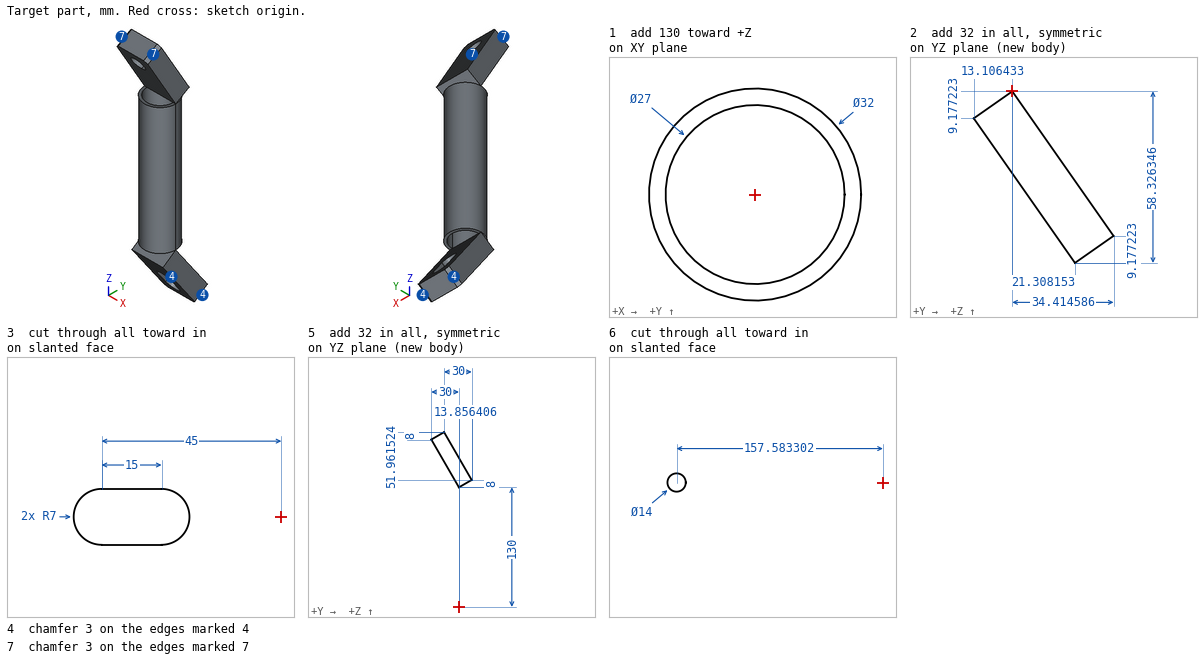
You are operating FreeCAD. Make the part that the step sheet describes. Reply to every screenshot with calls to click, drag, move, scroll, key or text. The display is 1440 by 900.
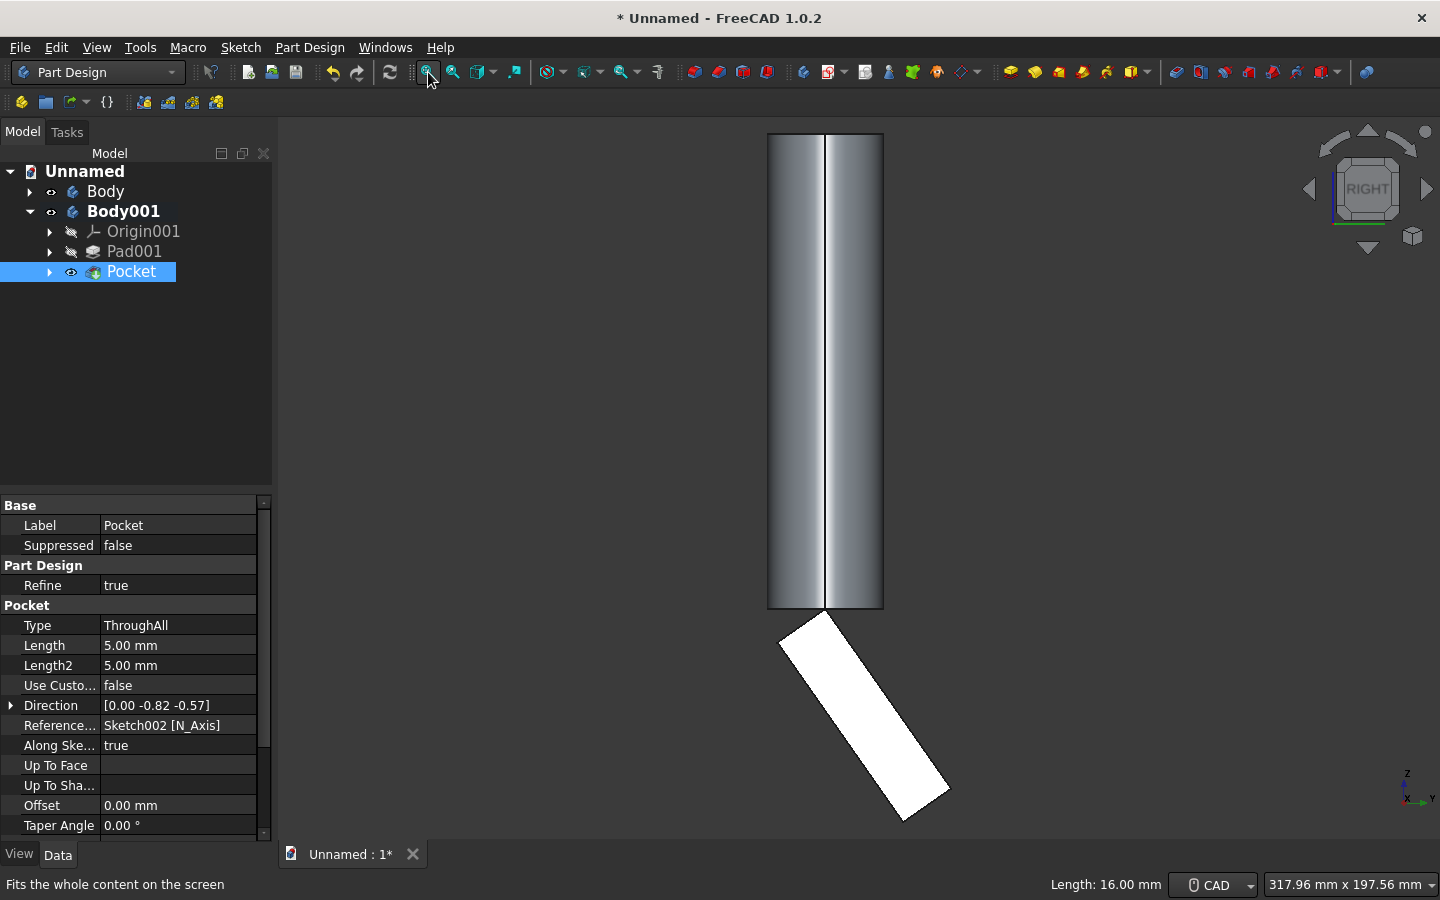
click(927, 804, ctrl)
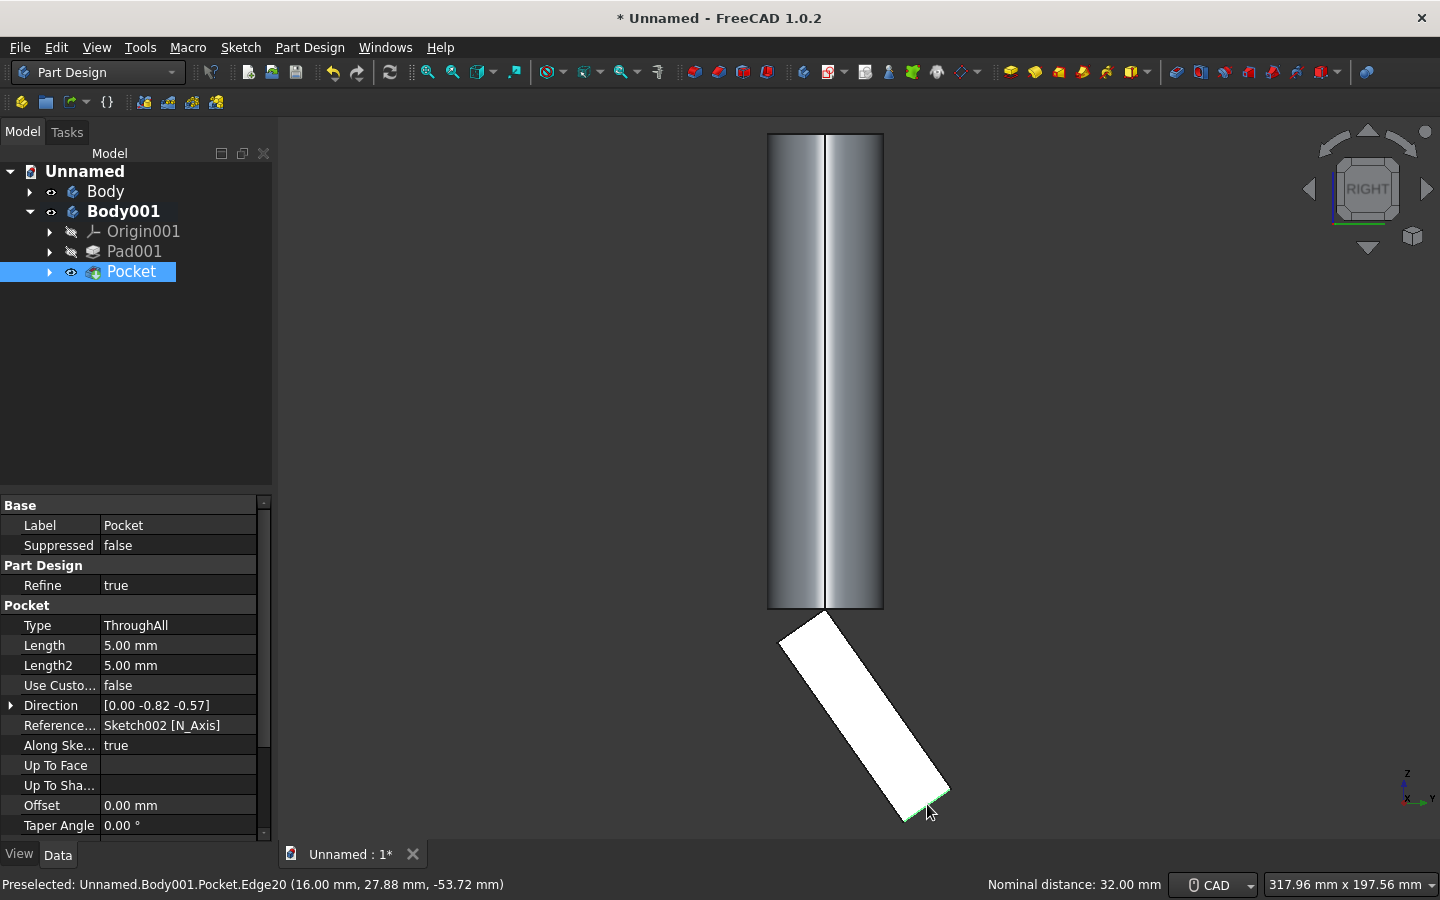
click(720, 72)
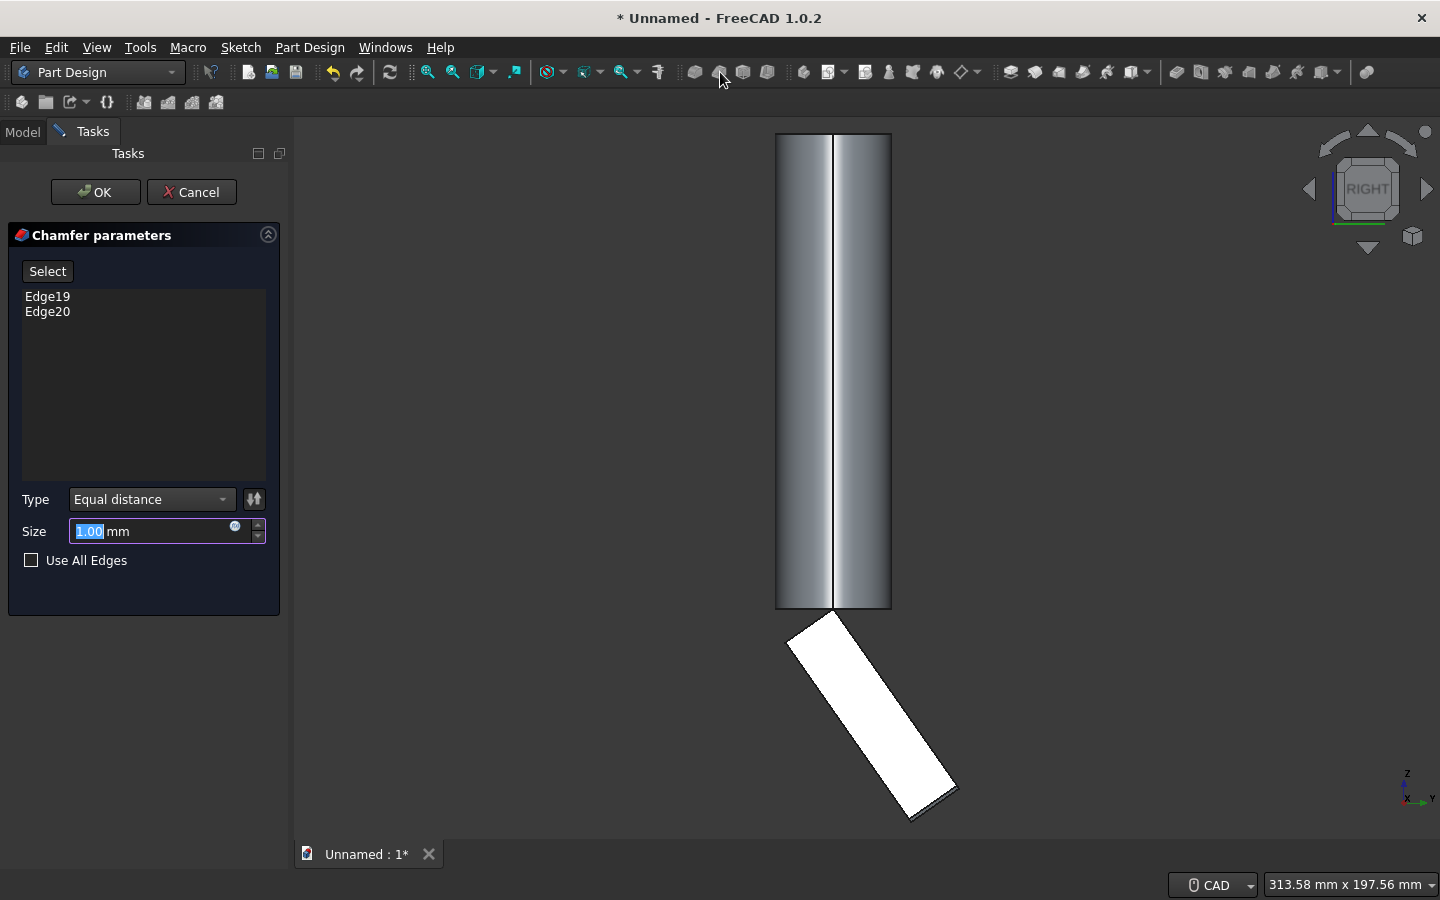
text(3)
key(Tab)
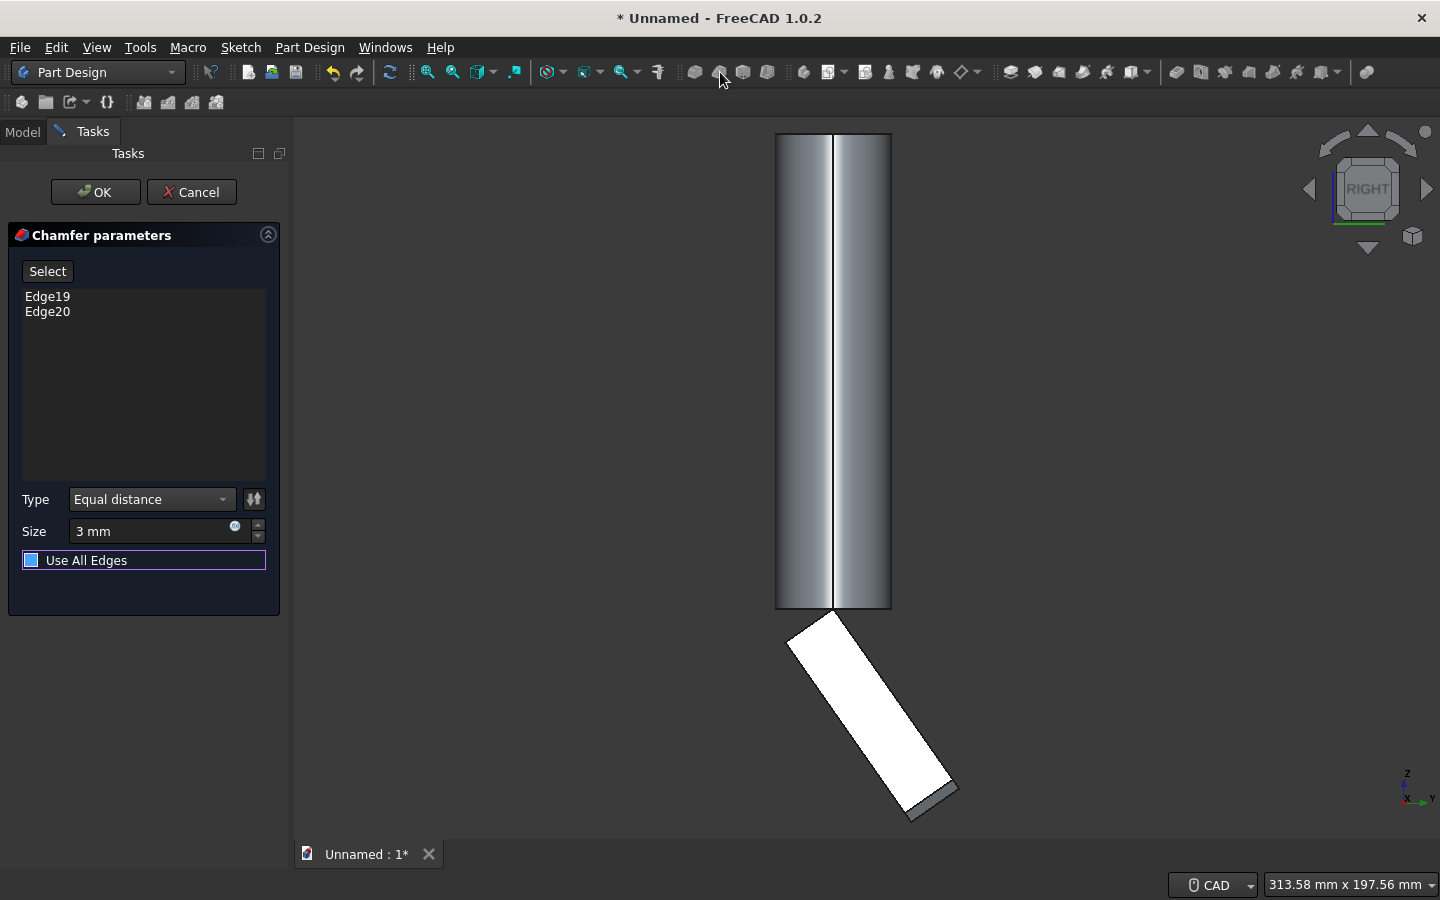
click(96, 192)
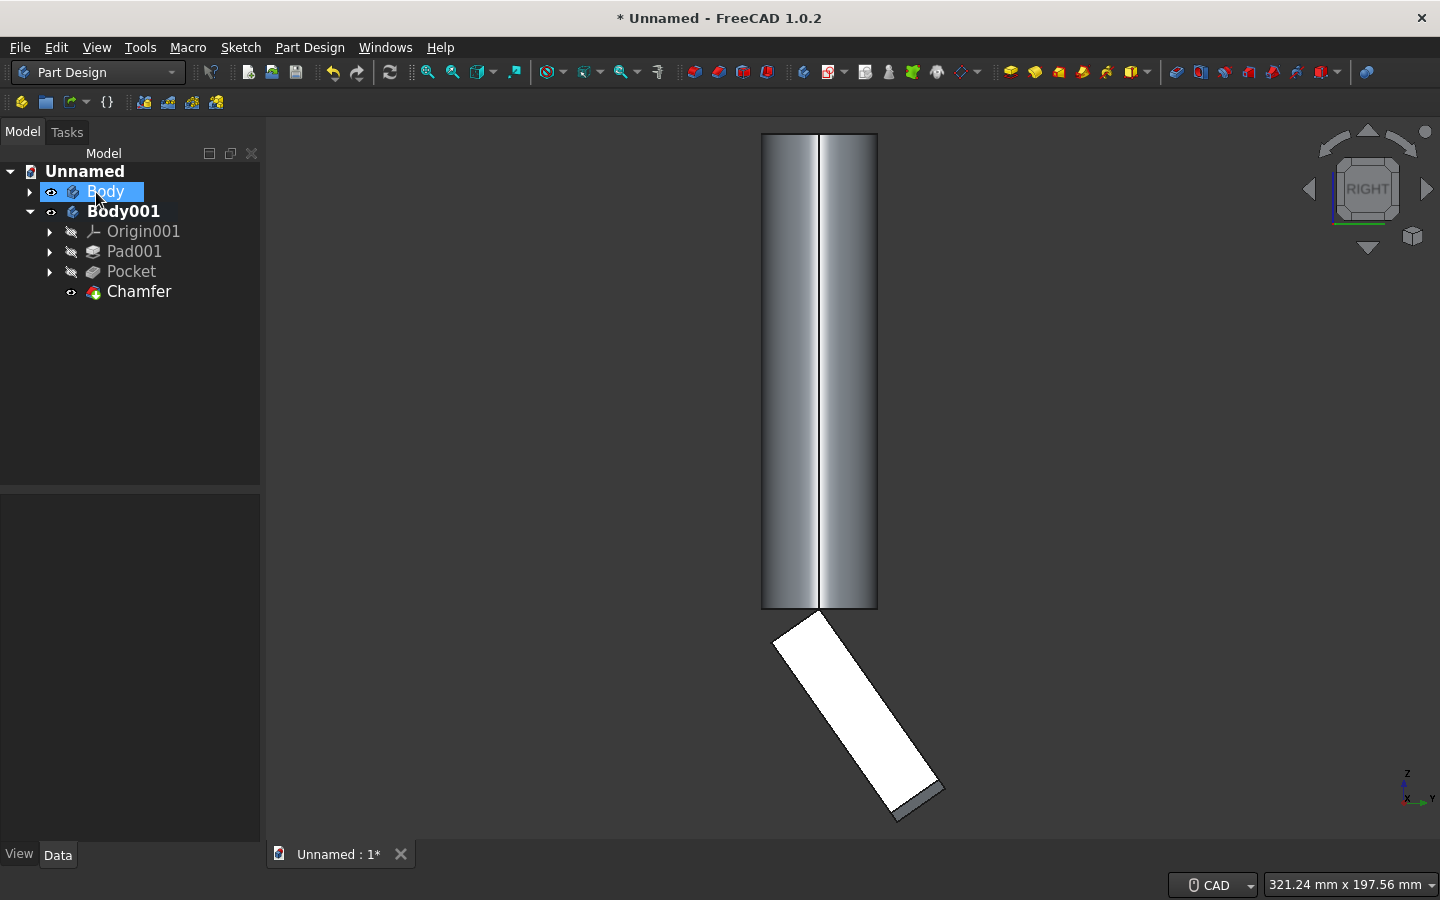
key(v)
key(f)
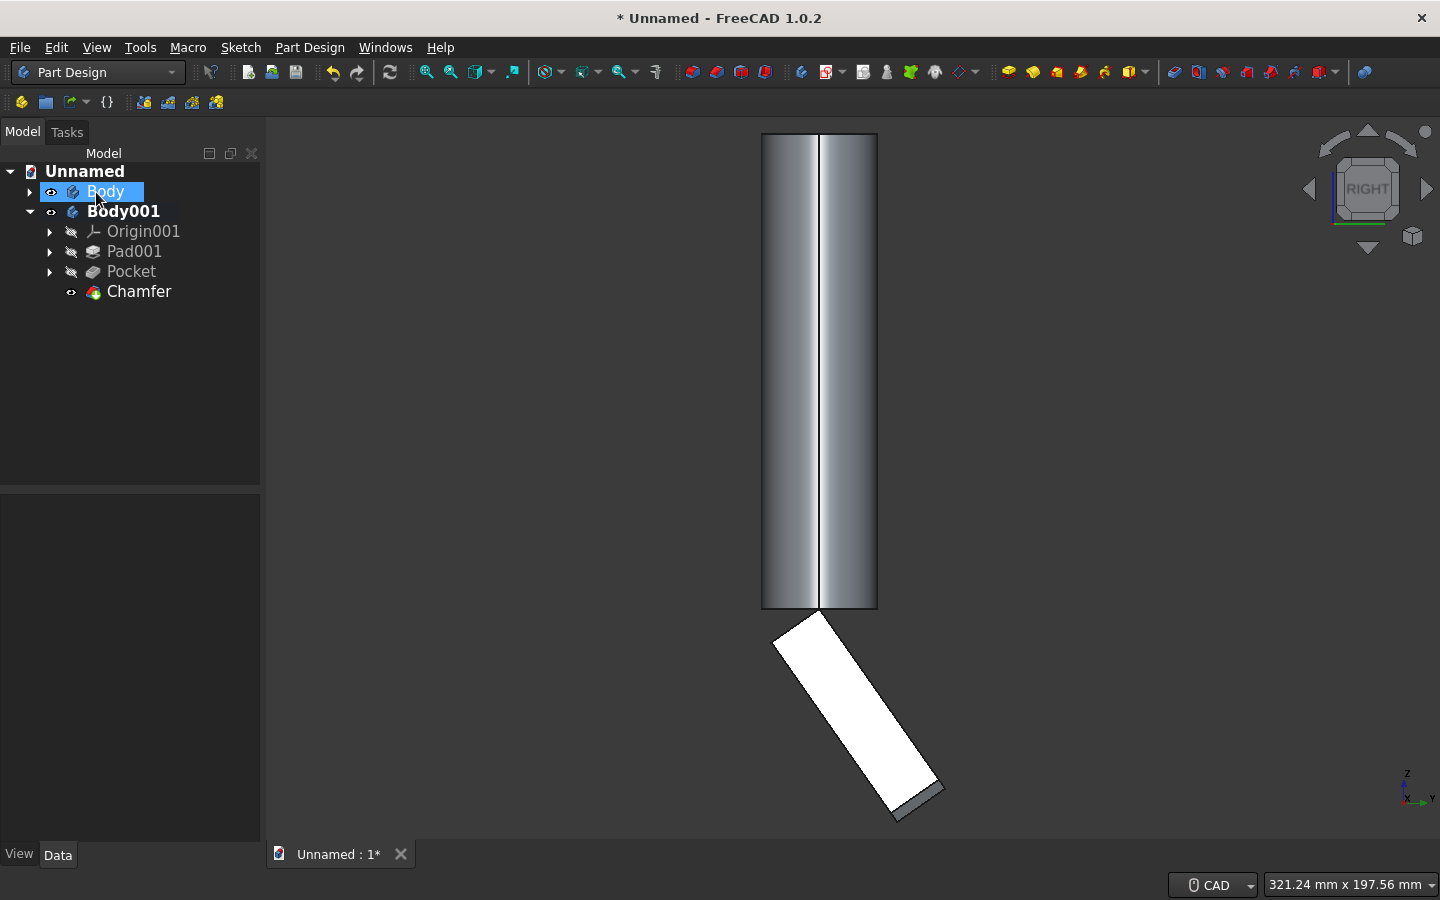
click(802, 72)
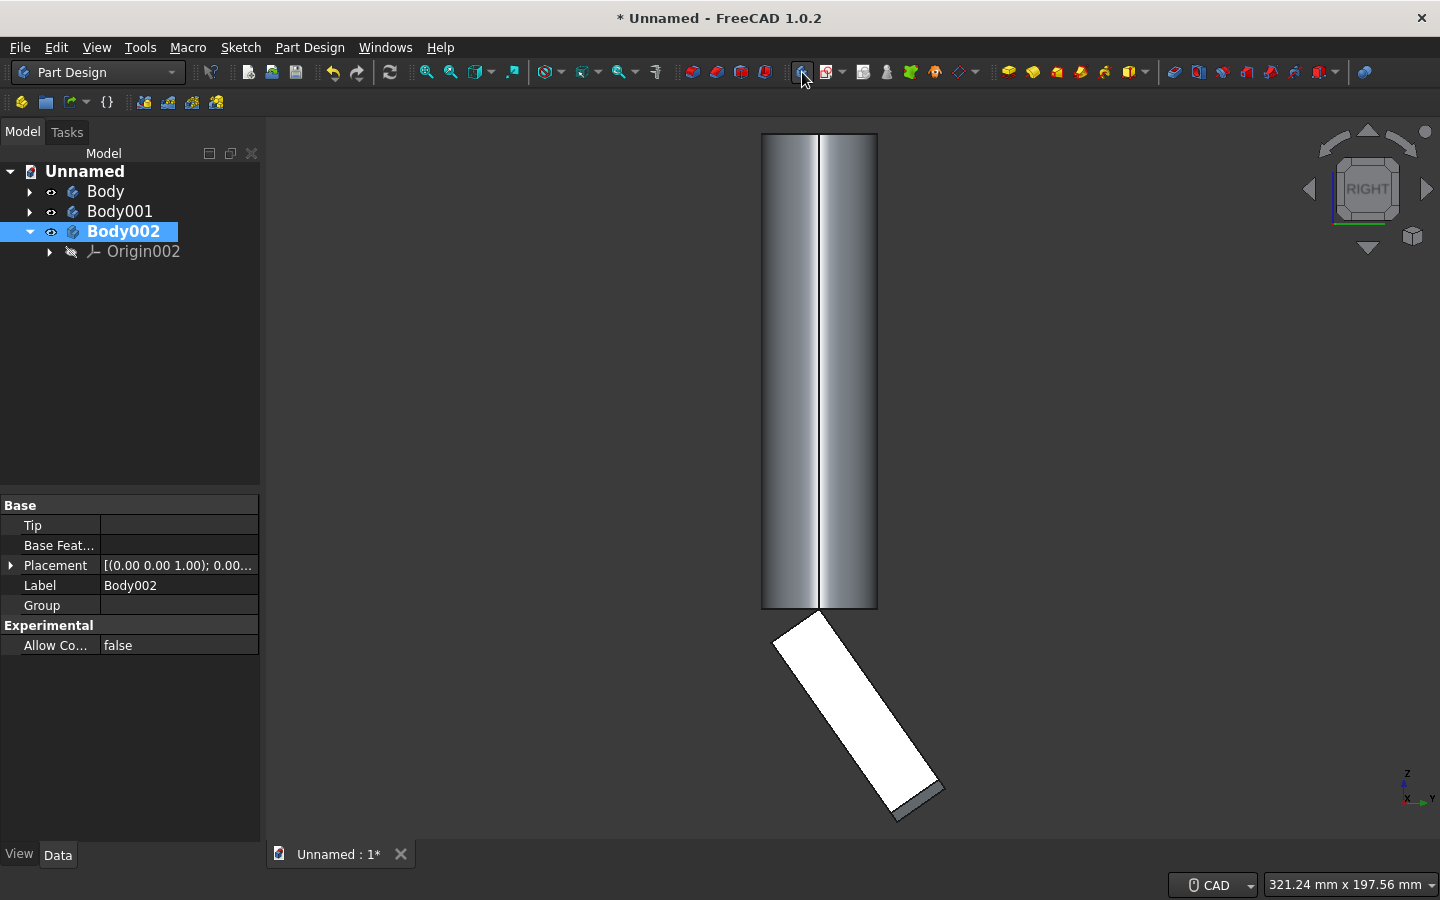
click(306, 799)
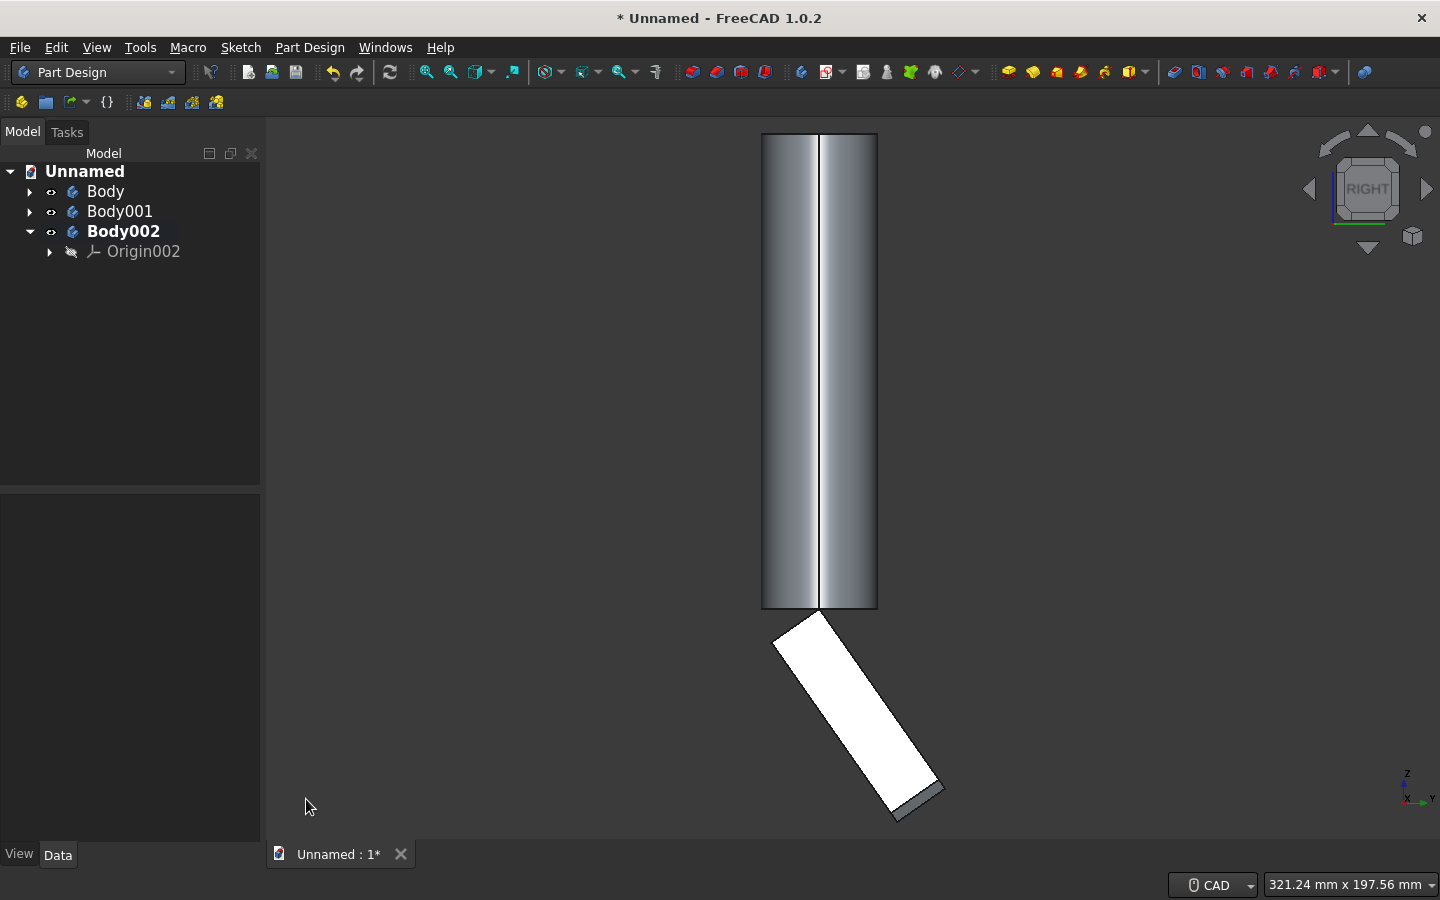
click(826, 72)